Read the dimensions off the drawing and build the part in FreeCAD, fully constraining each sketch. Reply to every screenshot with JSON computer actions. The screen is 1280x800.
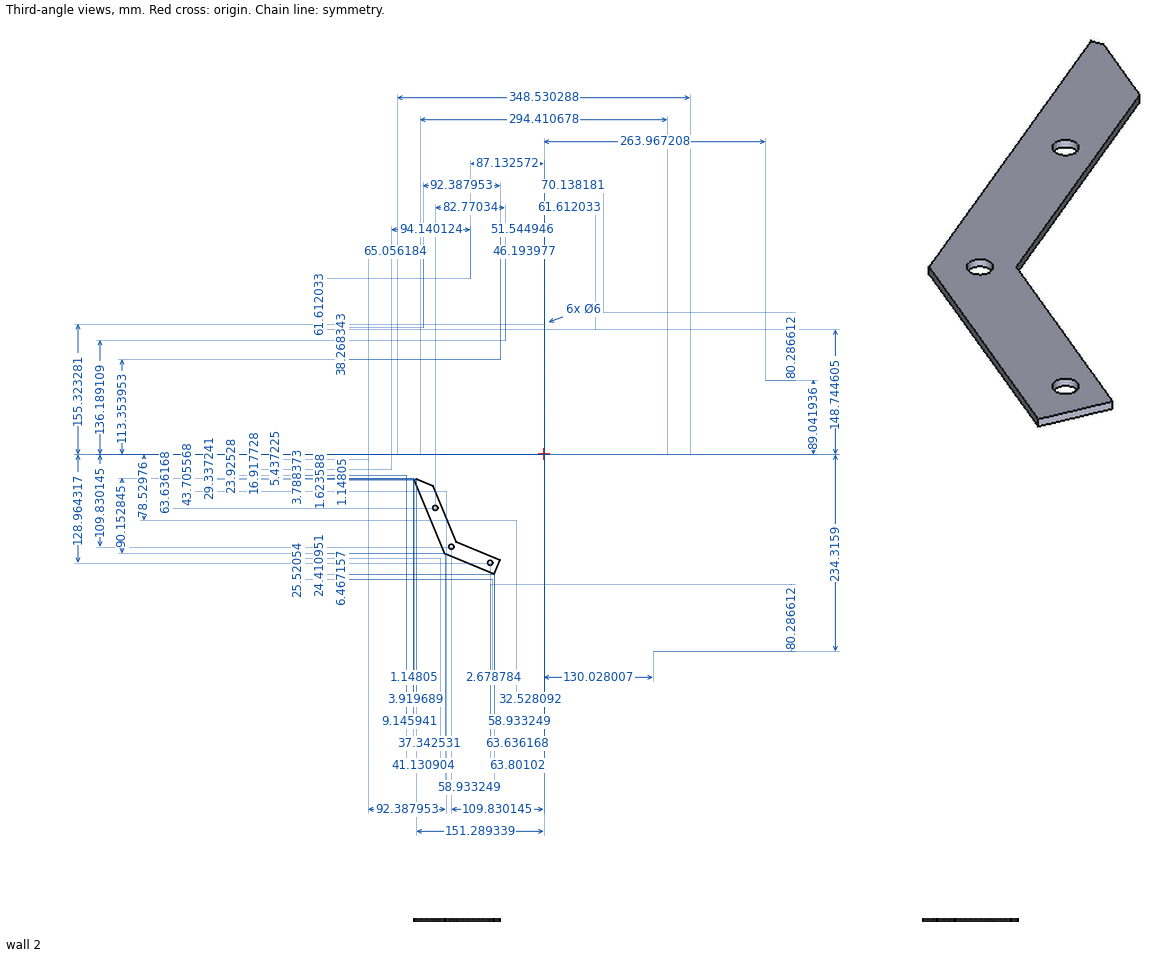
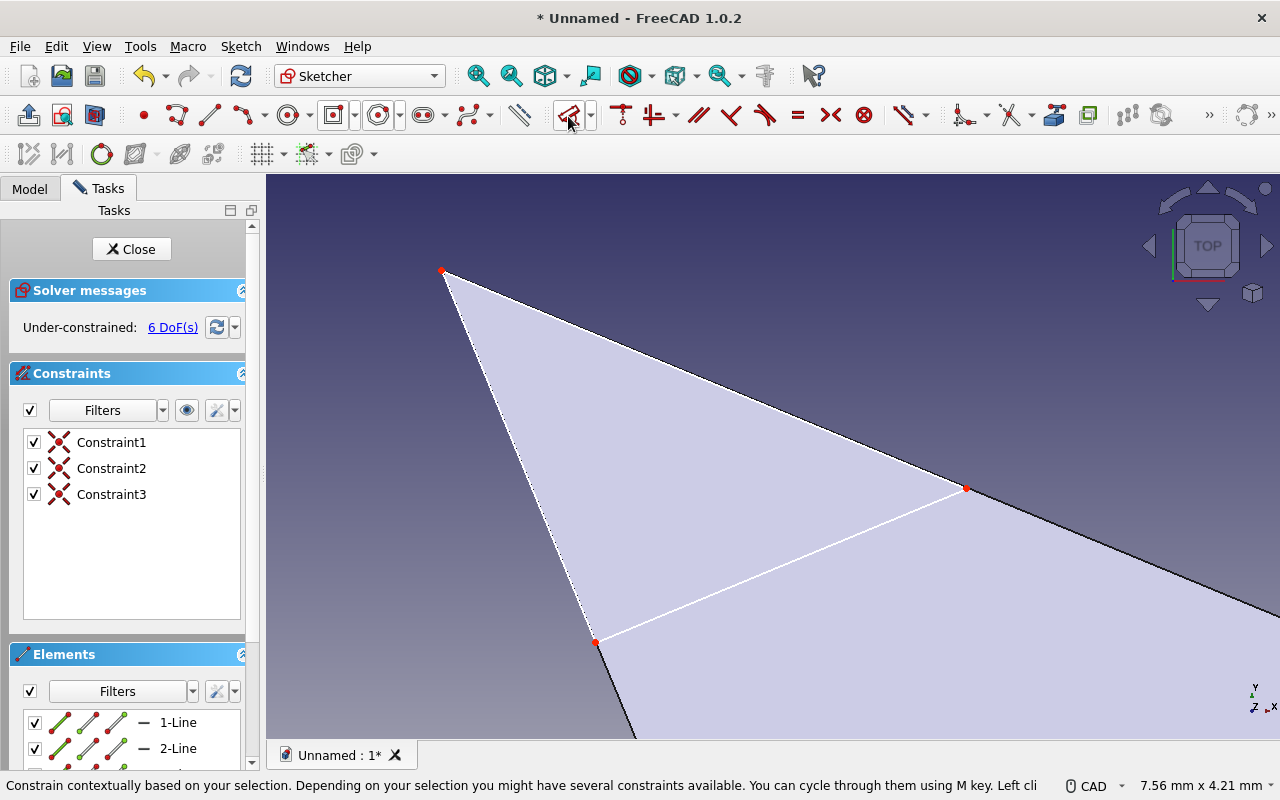
{"action": "left_click", "coordinate": [488, 383]}
{"action": "left_click", "coordinate": [519, 677]}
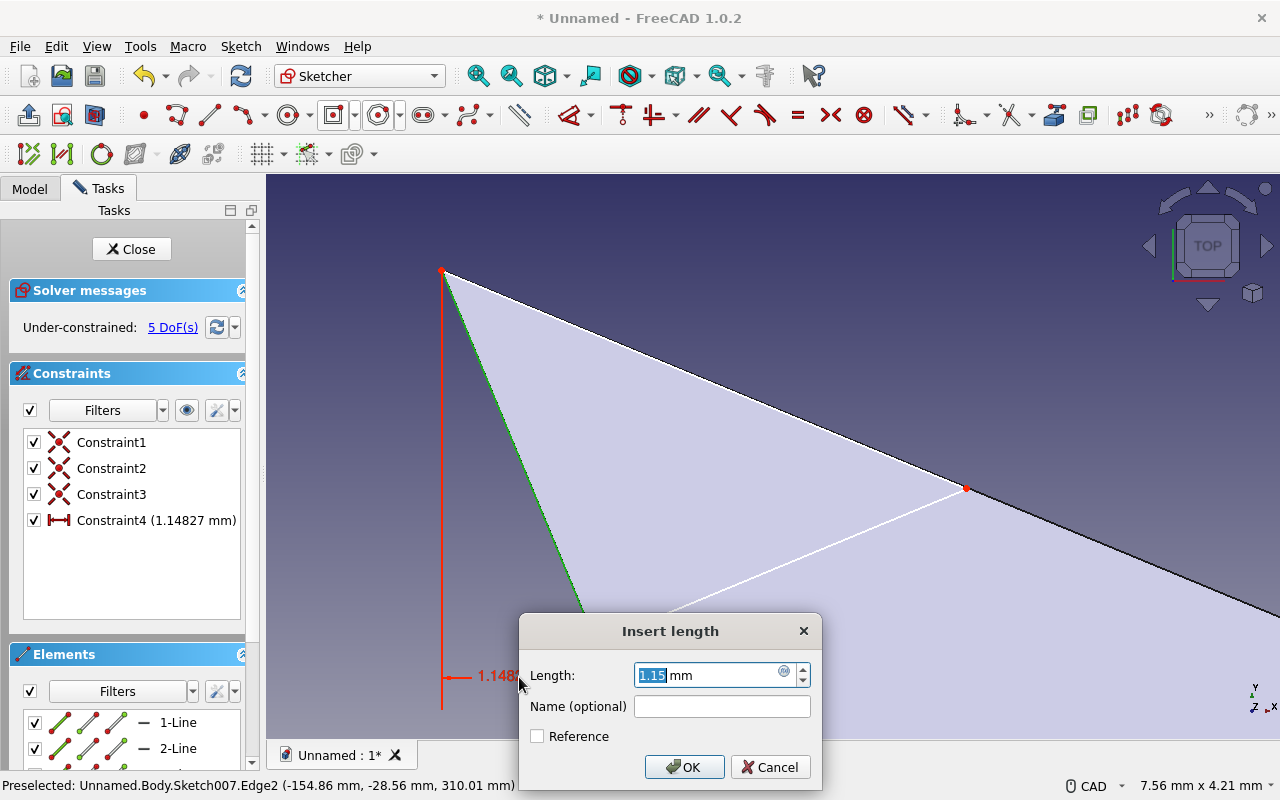
{"action": "type", "text": "1.14805"}
{"action": "key", "text": "Return"}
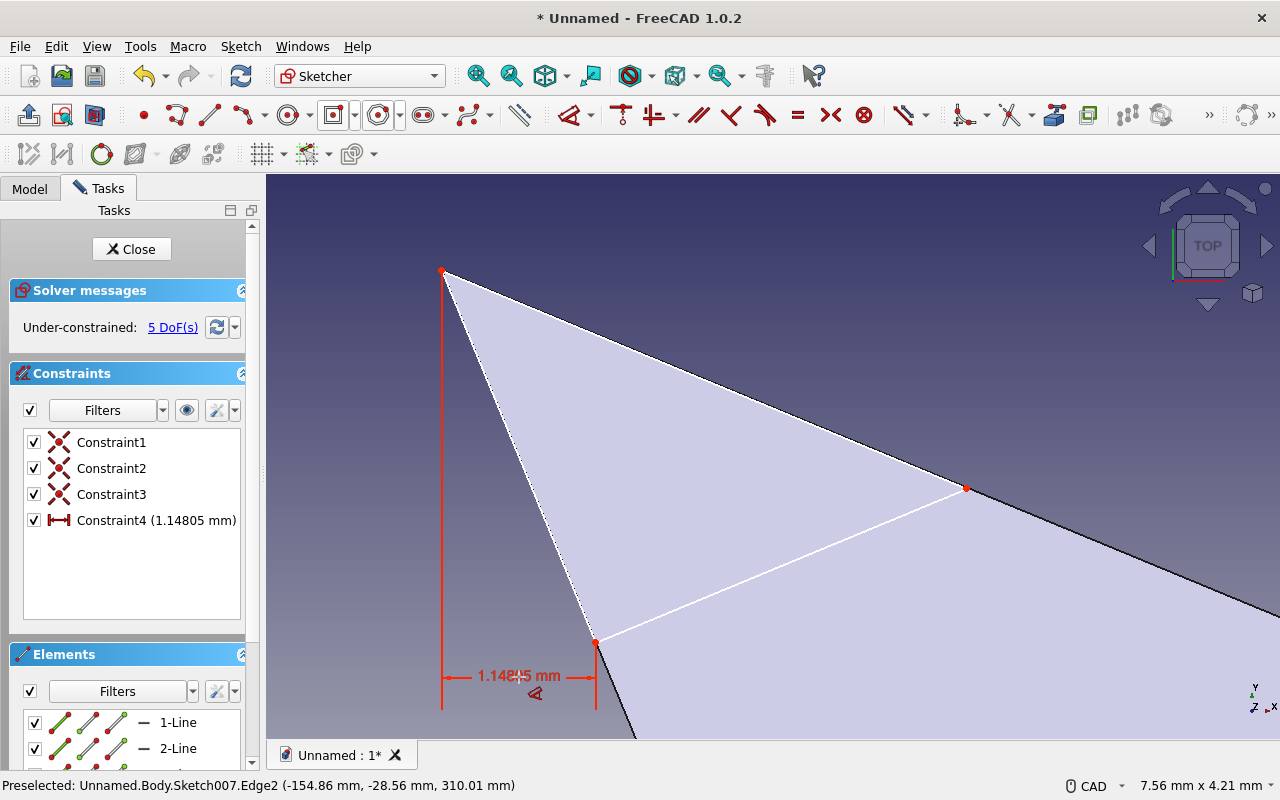
{"action": "left_click", "coordinate": [707, 597]}
{"action": "left_click", "coordinate": [1001, 566]}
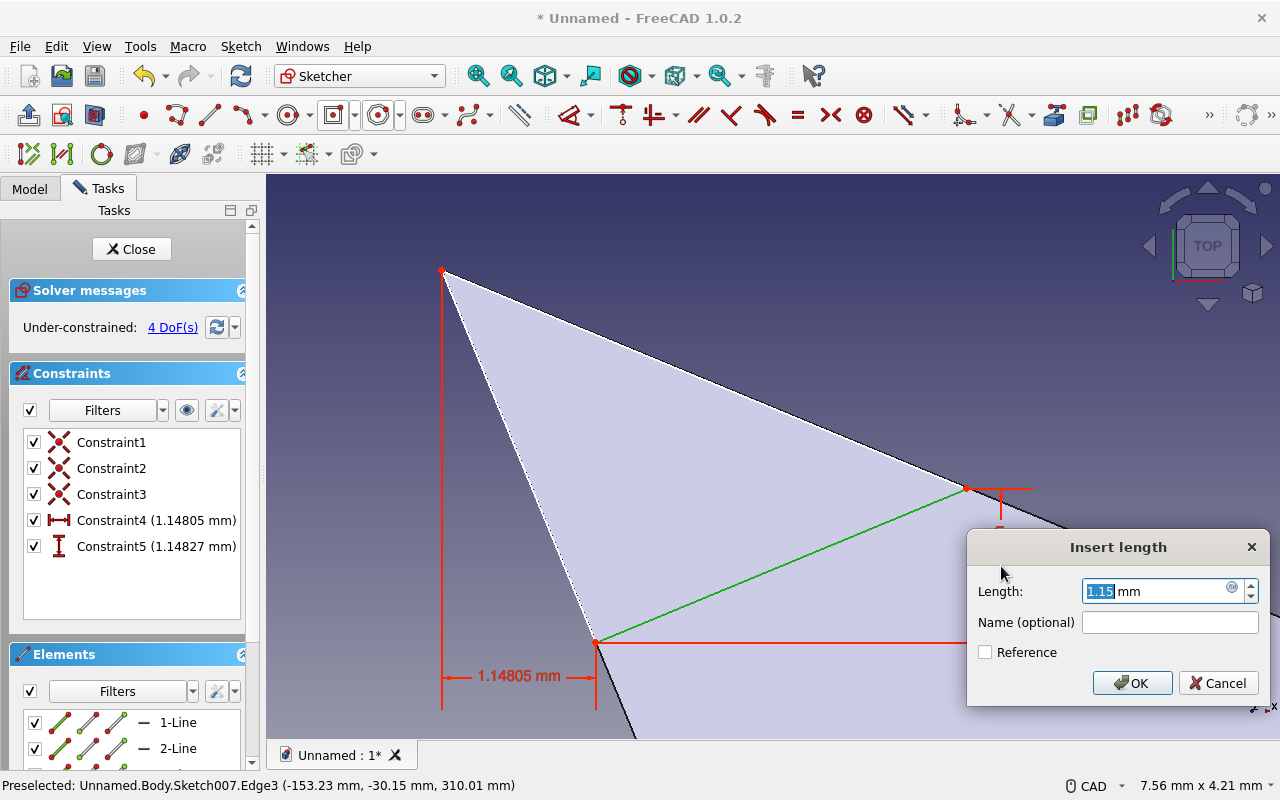
{"action": "type", "text": "1.14805"}
{"action": "key", "text": "Return"}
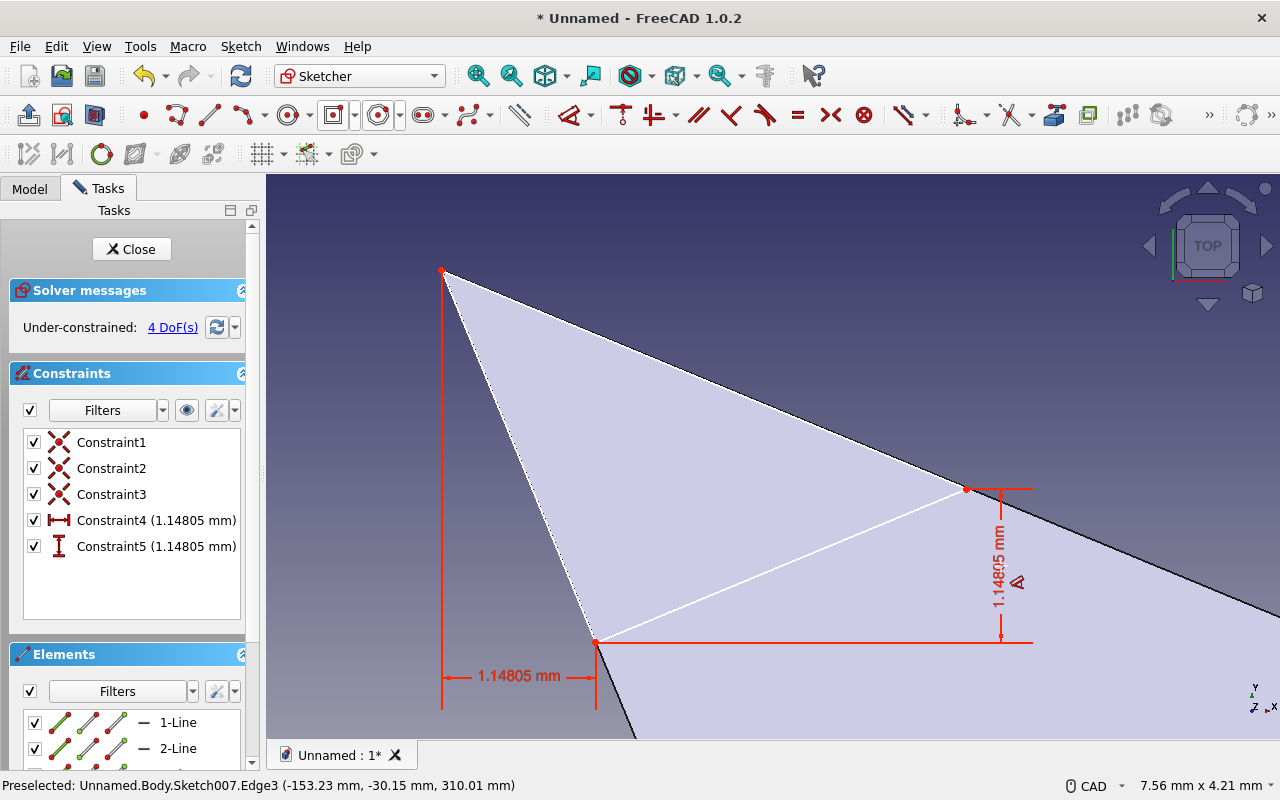
{"action": "left_click", "coordinate": [809, 424]}
{"action": "left_click", "coordinate": [704, 237]}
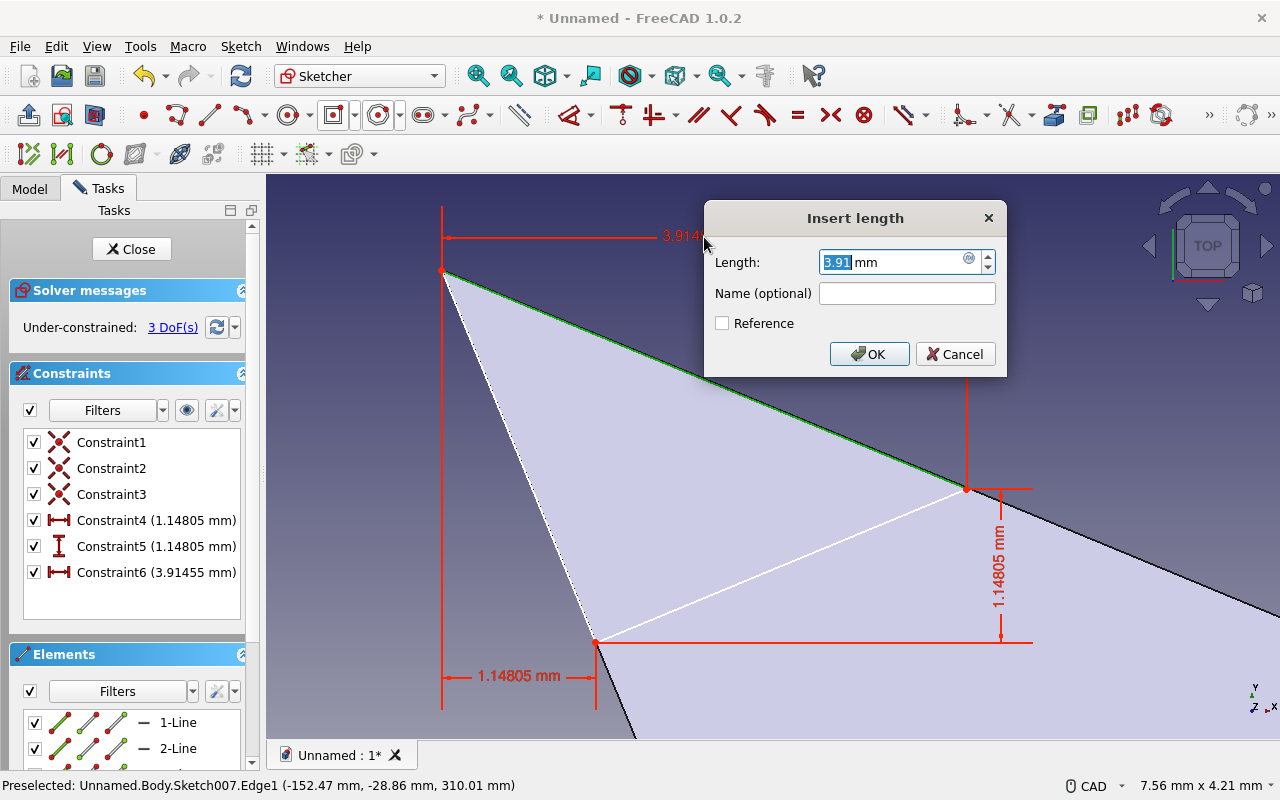
{"action": "type", "text": "3.919689"}
{"action": "key", "text": "Return"}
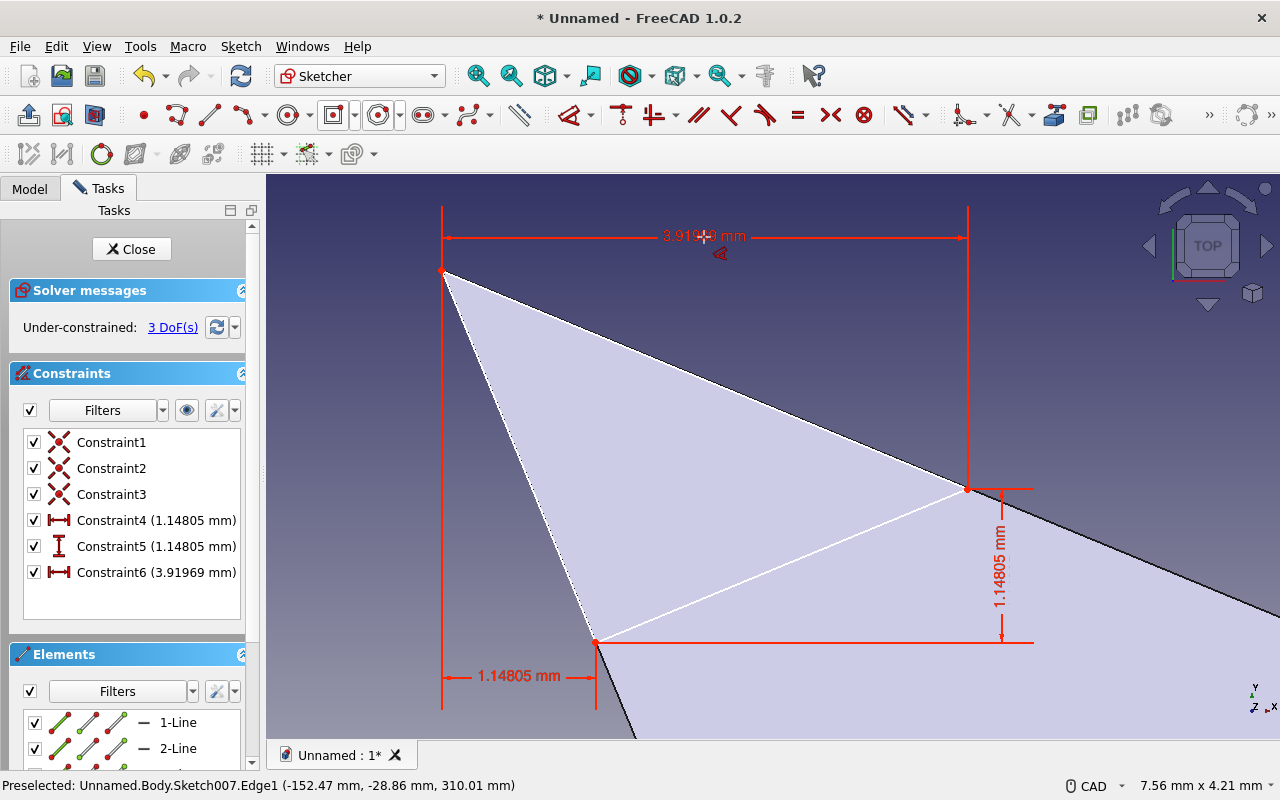
{"action": "left_click", "coordinate": [810, 424]}
{"action": "left_click", "coordinate": [1002, 380]}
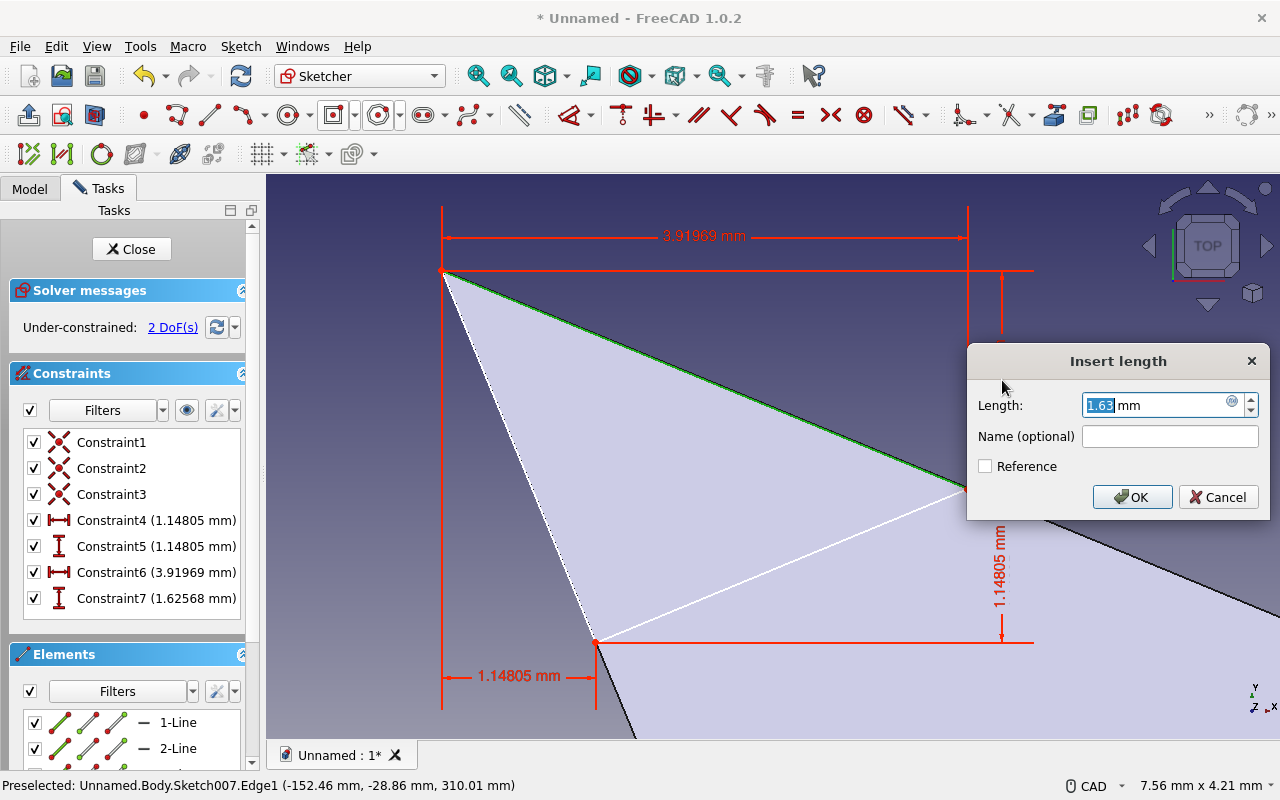
{"action": "type", "text": "1.623588"}
{"action": "key", "text": "Return"}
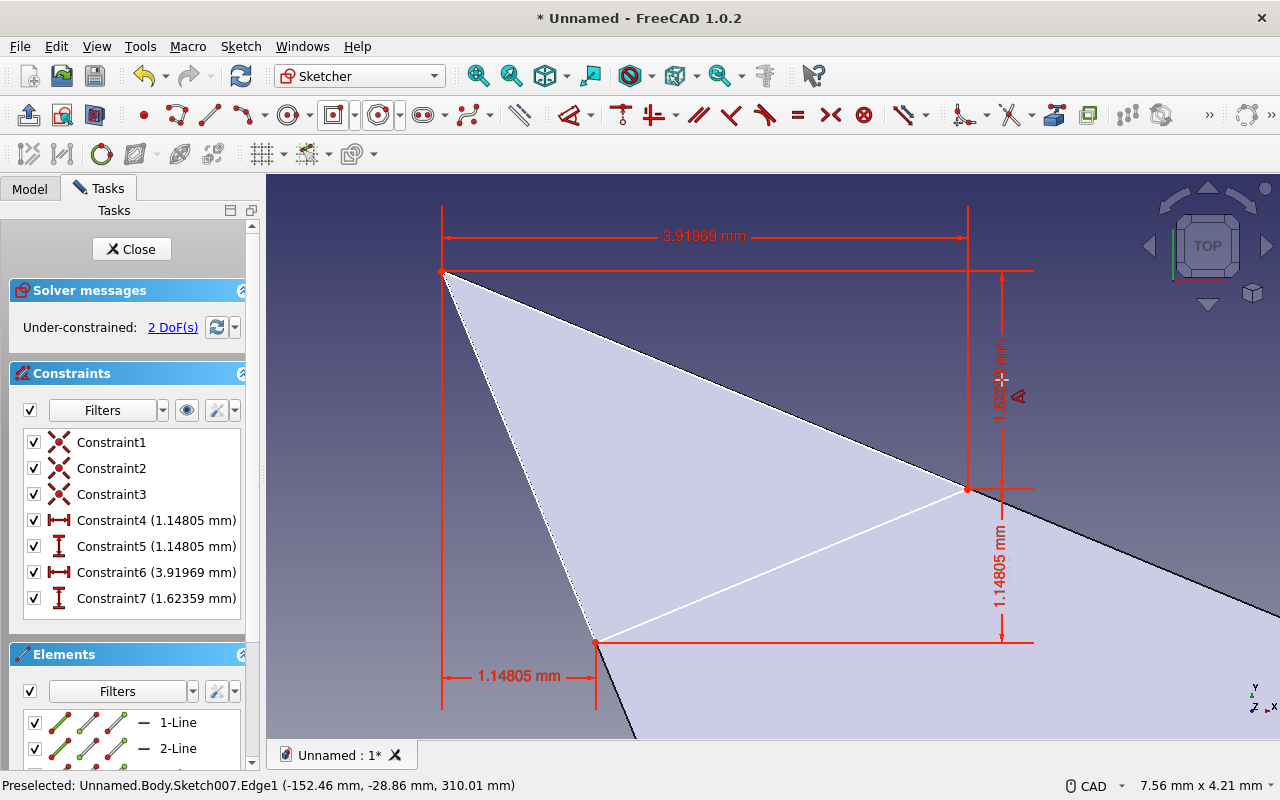
{"action": "left_click", "coordinate": [968, 489]}
{"action": "left_click", "coordinate": [934, 346]}